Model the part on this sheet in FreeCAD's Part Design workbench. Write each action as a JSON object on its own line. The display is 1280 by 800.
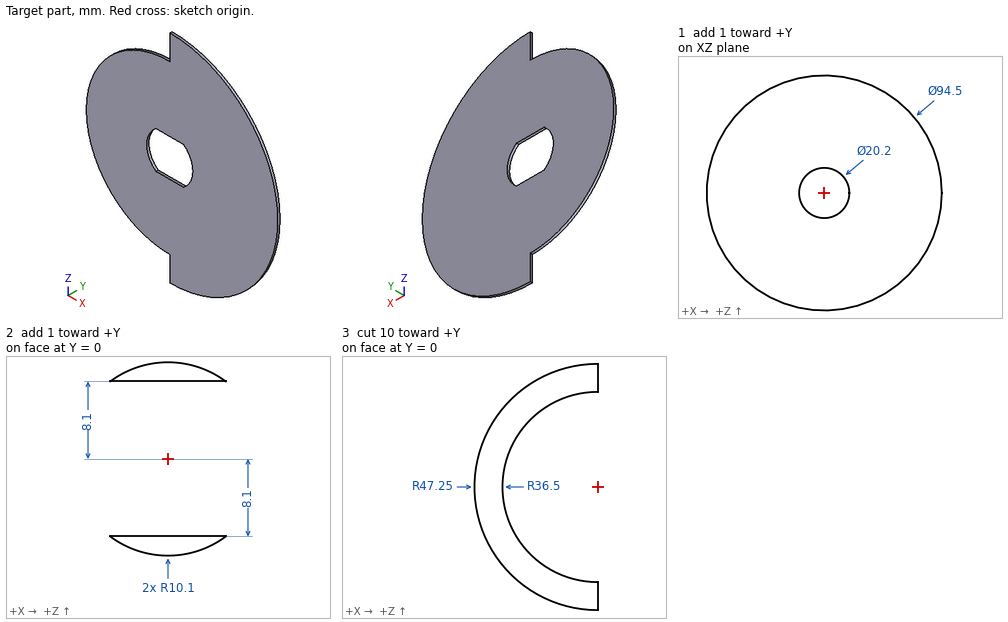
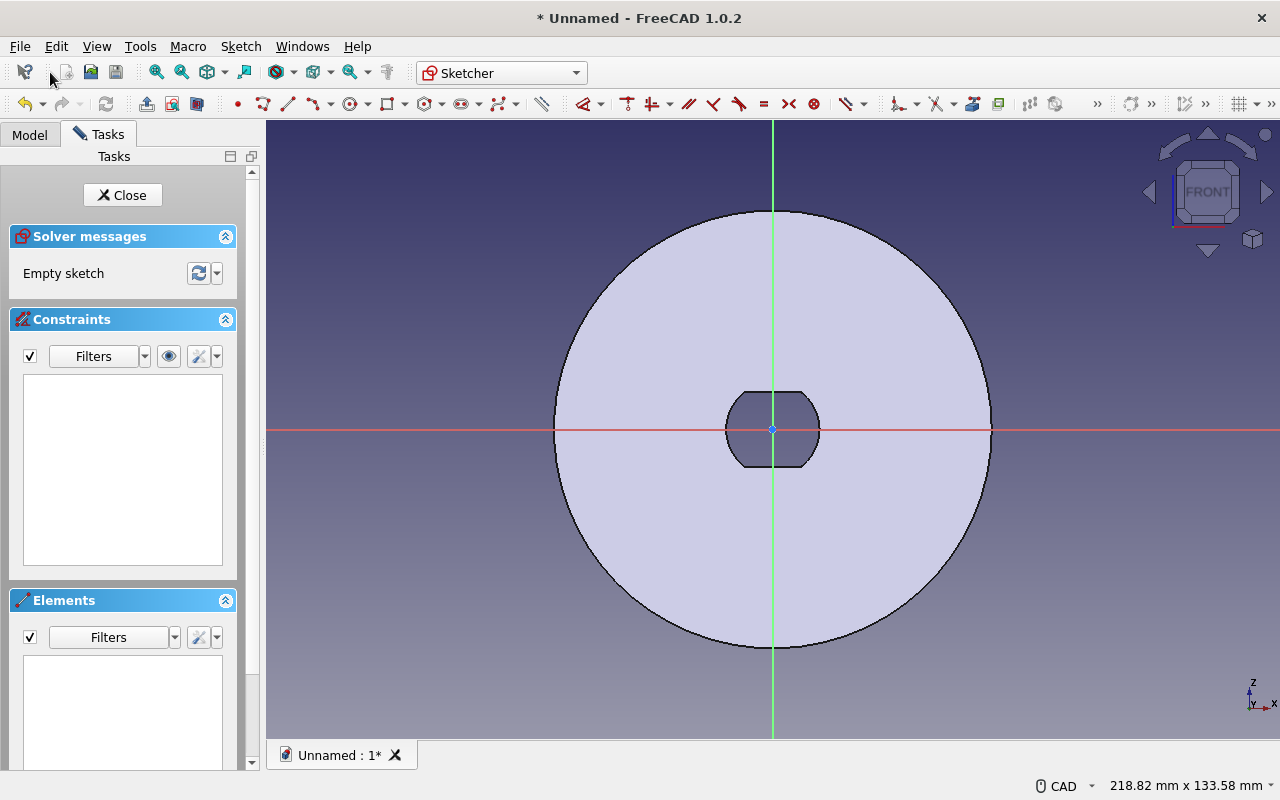
{"action": "left_click", "coordinate": [288, 104]}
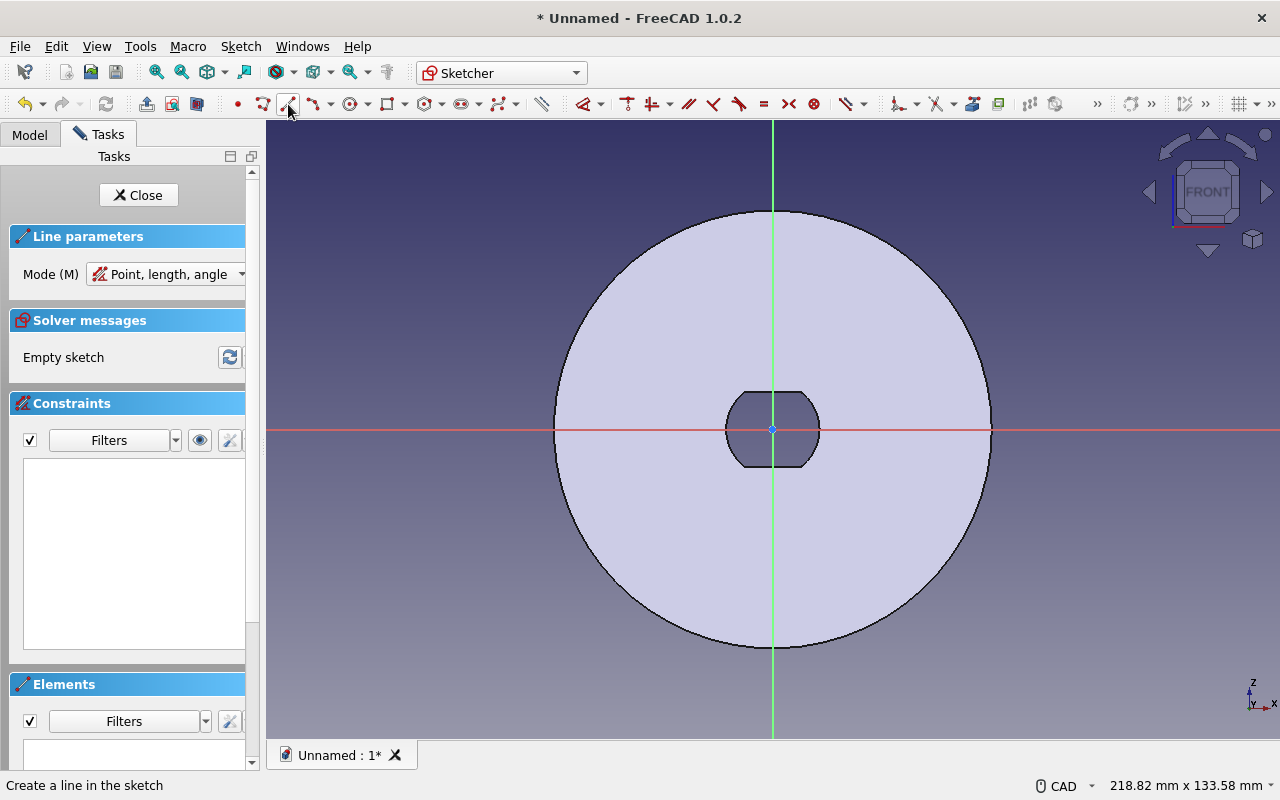
{"action": "left_click", "coordinate": [773, 260]}
{"action": "left_click", "coordinate": [764, 211]}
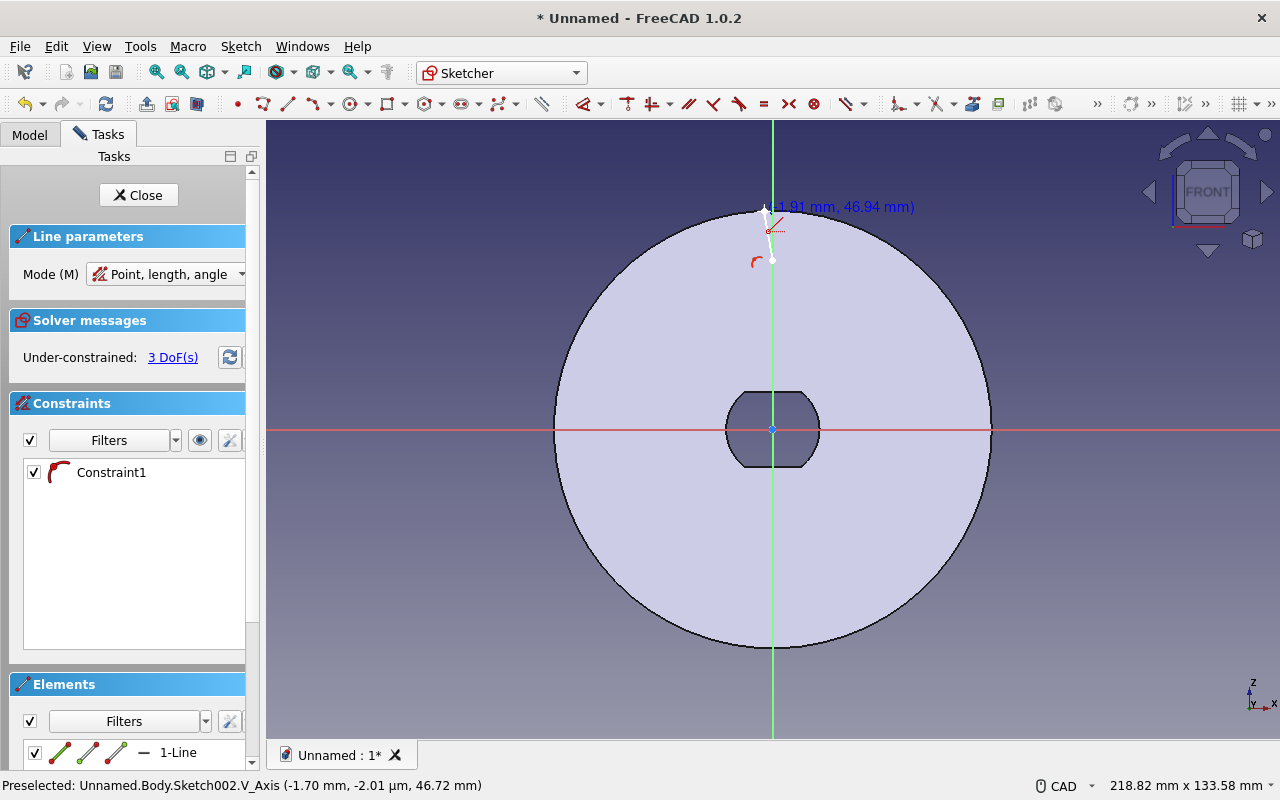
{"action": "left_click", "coordinate": [773, 648]}
{"action": "left_click", "coordinate": [764, 599]}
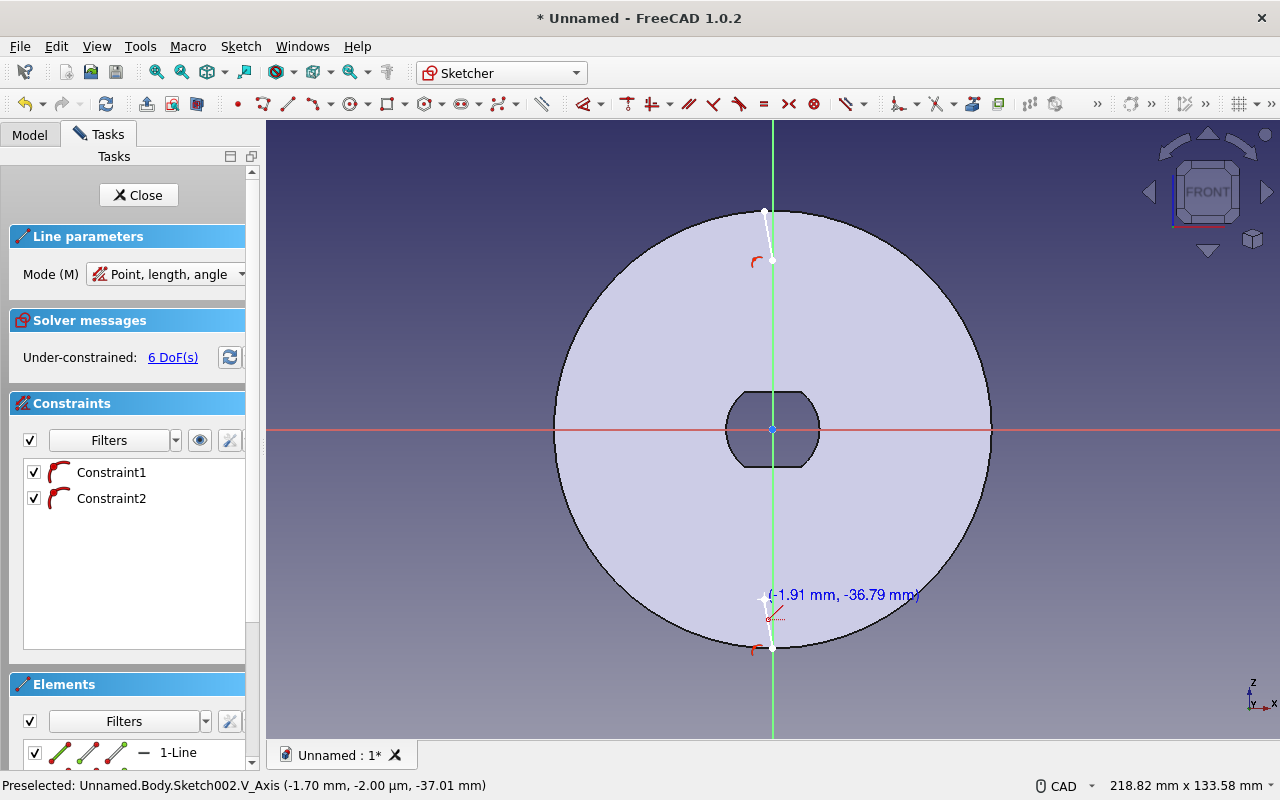
{"action": "left_click", "coordinate": [312, 104]}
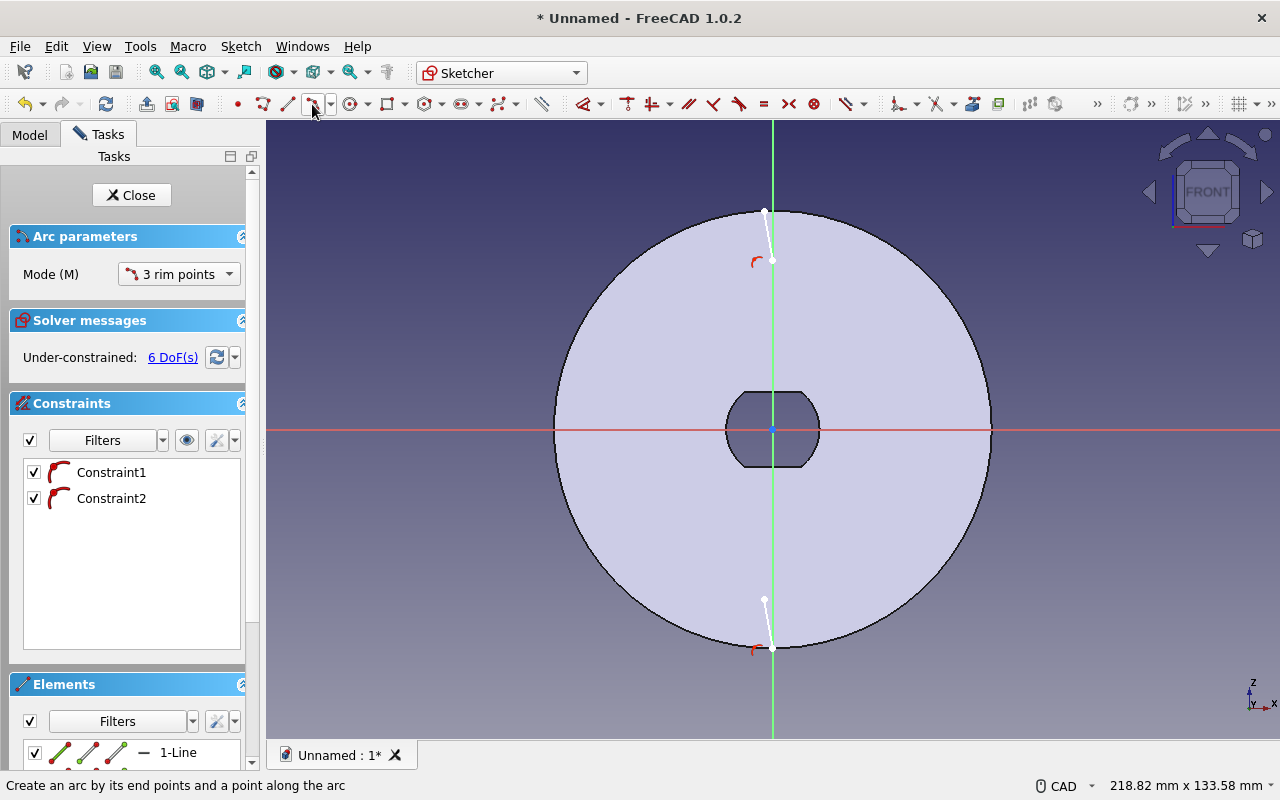
{"action": "left_click", "coordinate": [764, 212]}
{"action": "left_click", "coordinate": [773, 649]}
{"action": "left_click", "coordinate": [565, 362]}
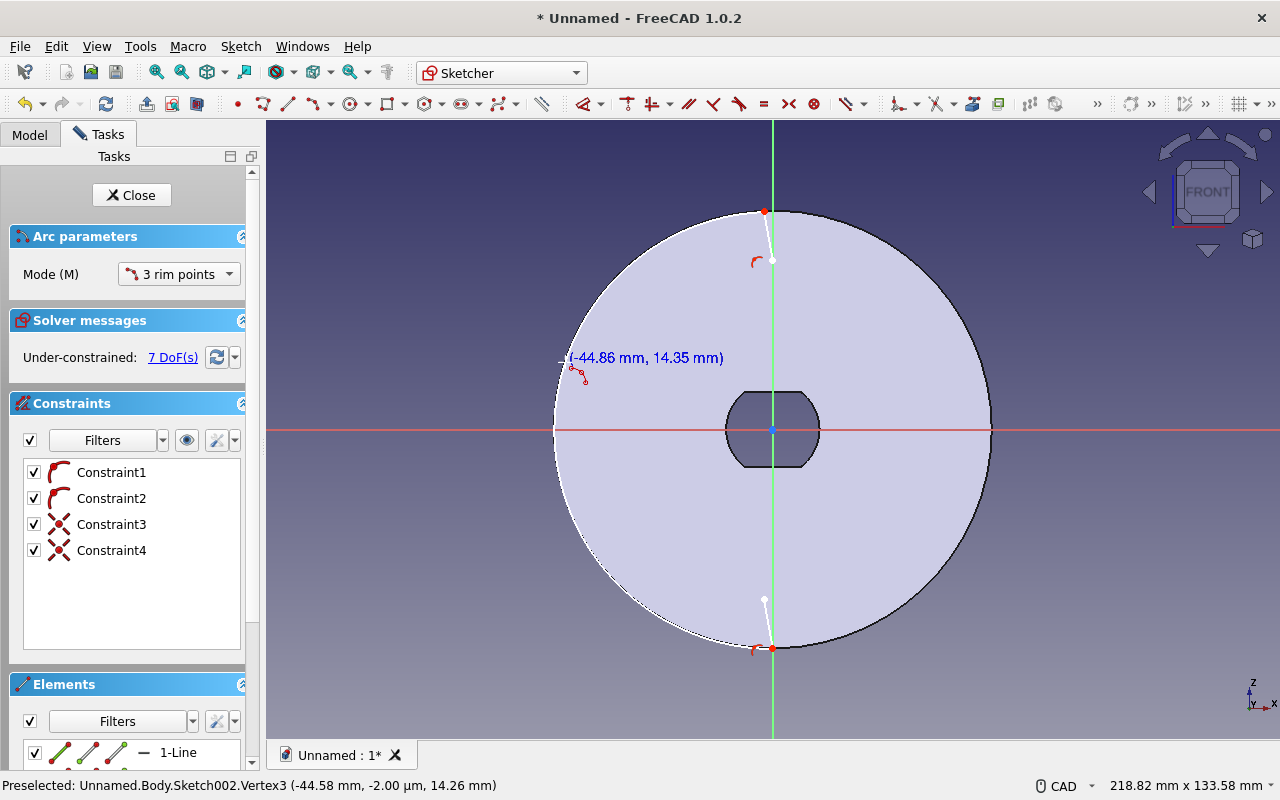
{"action": "left_click", "coordinate": [764, 600]}
{"action": "left_click", "coordinate": [773, 261]}
{"action": "left_click", "coordinate": [612, 377]}
{"action": "key", "text": "Escape"}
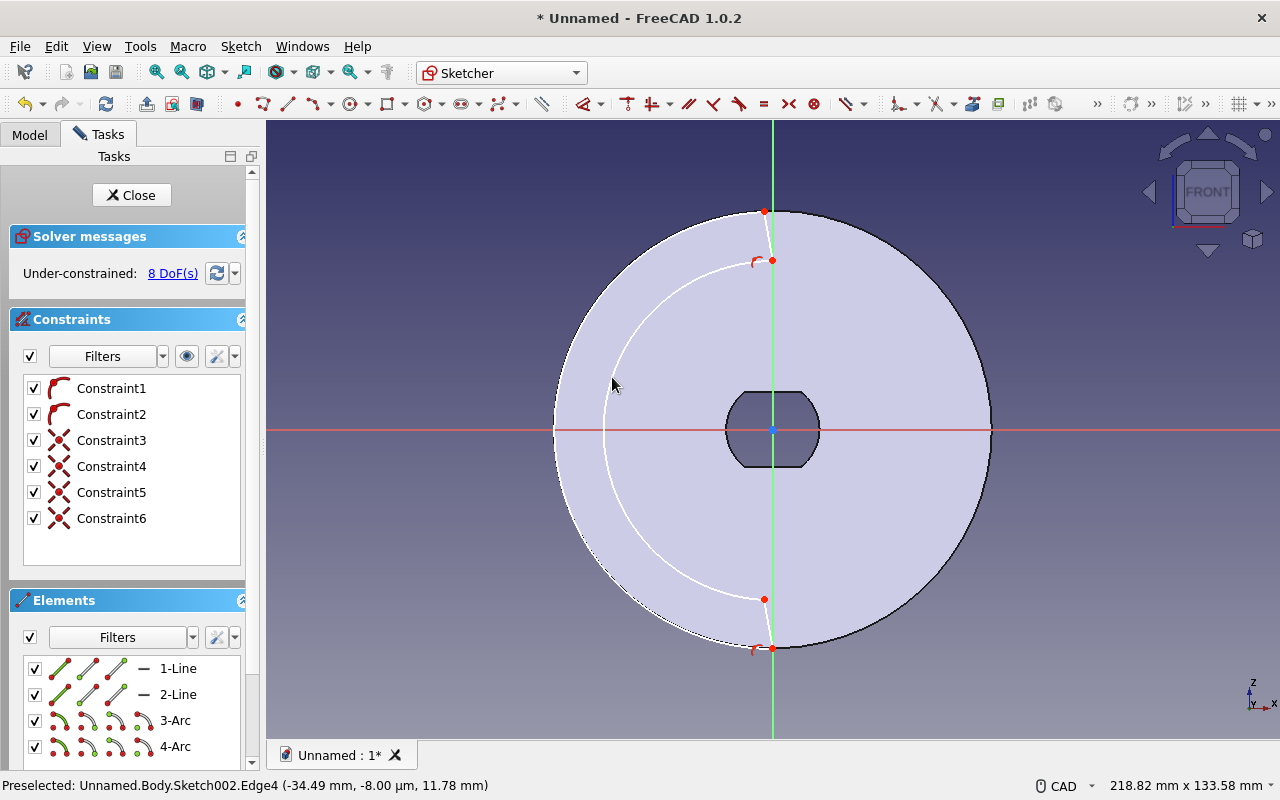
{"action": "left_click", "coordinate": [770, 246]}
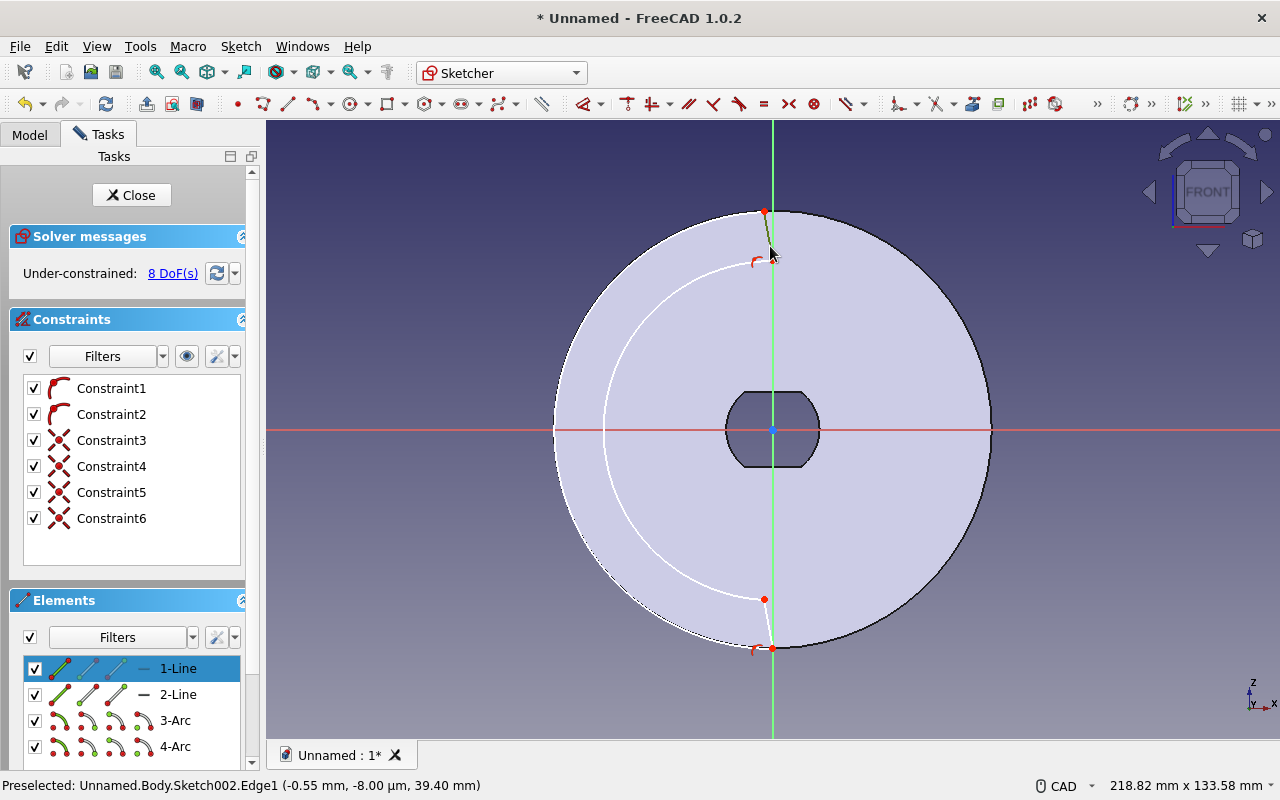
{"action": "left_click", "coordinate": [670, 104]}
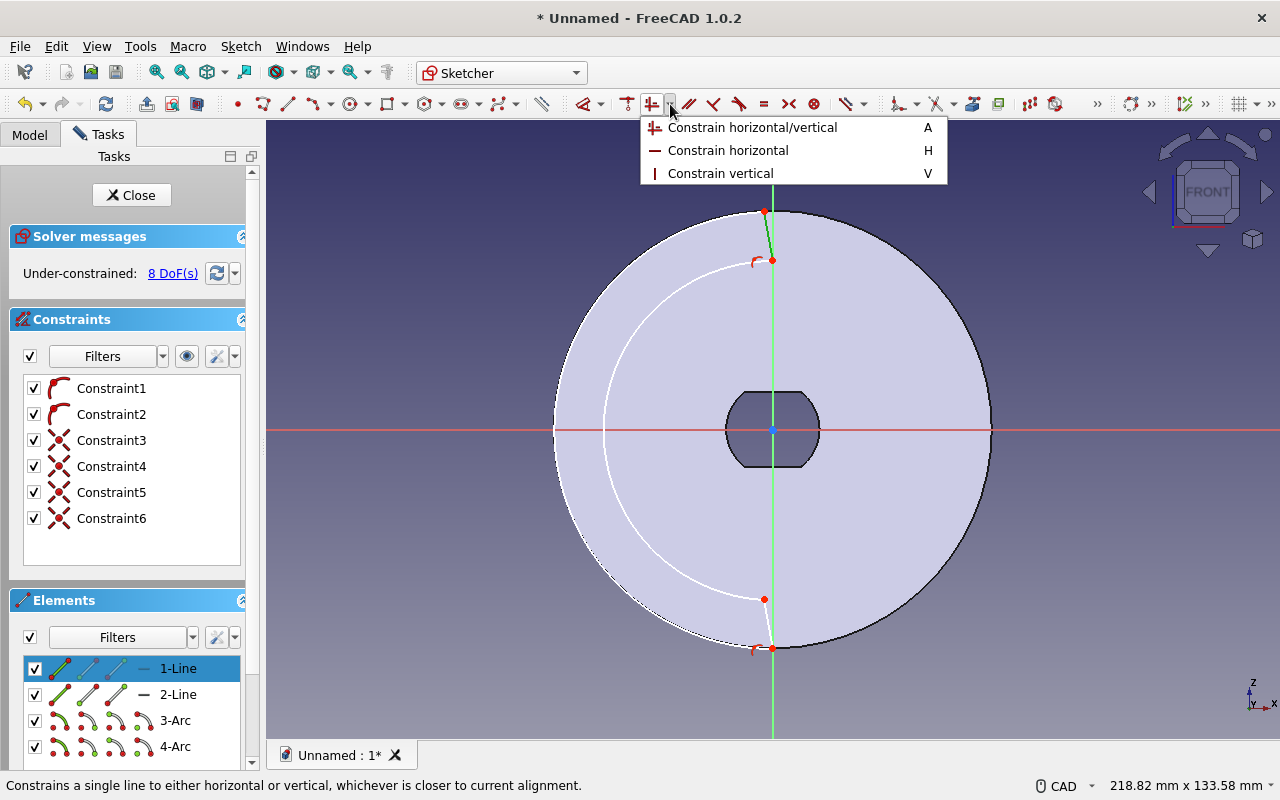
{"action": "left_click", "coordinate": [794, 174]}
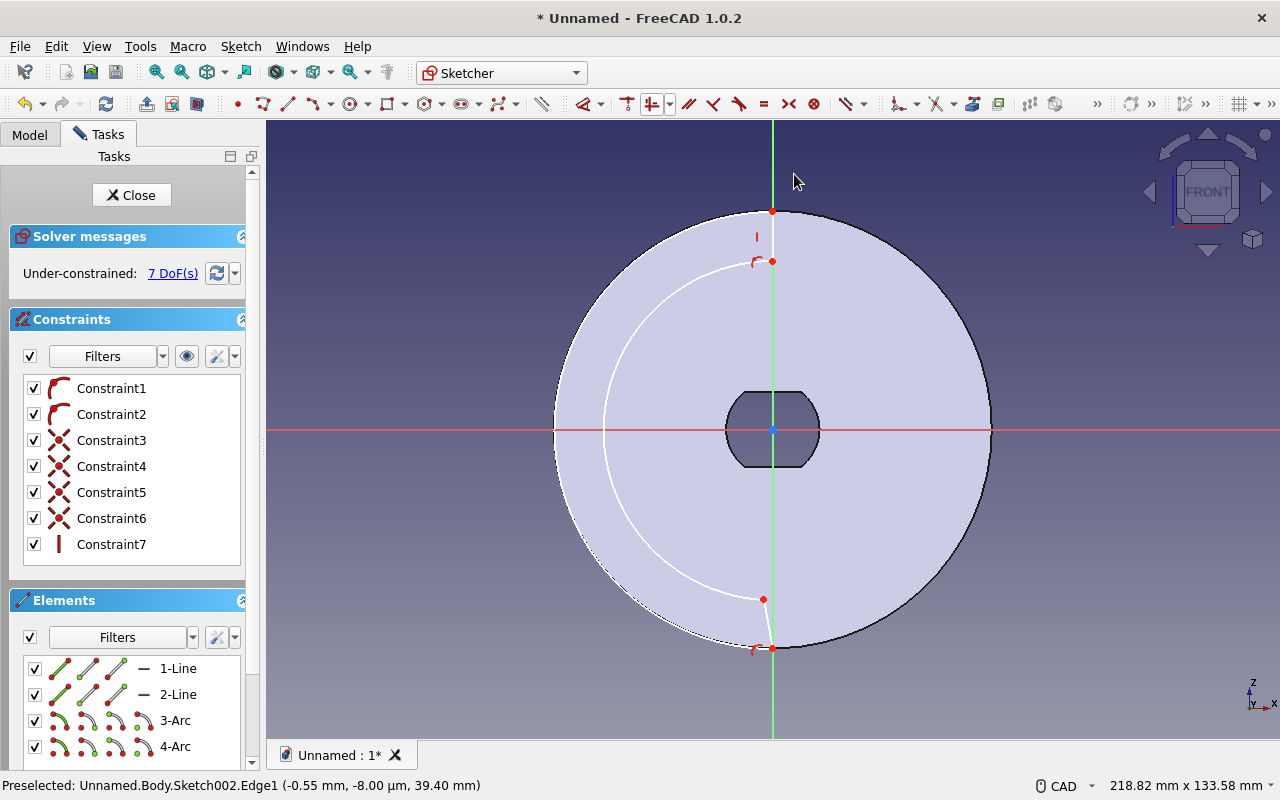
{"action": "left_click", "coordinate": [770, 634]}